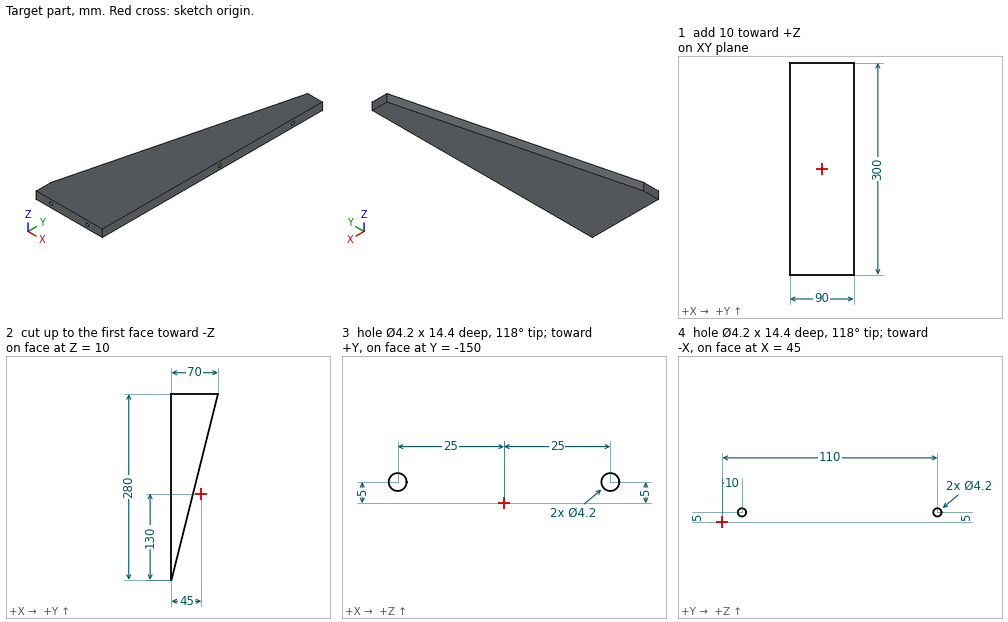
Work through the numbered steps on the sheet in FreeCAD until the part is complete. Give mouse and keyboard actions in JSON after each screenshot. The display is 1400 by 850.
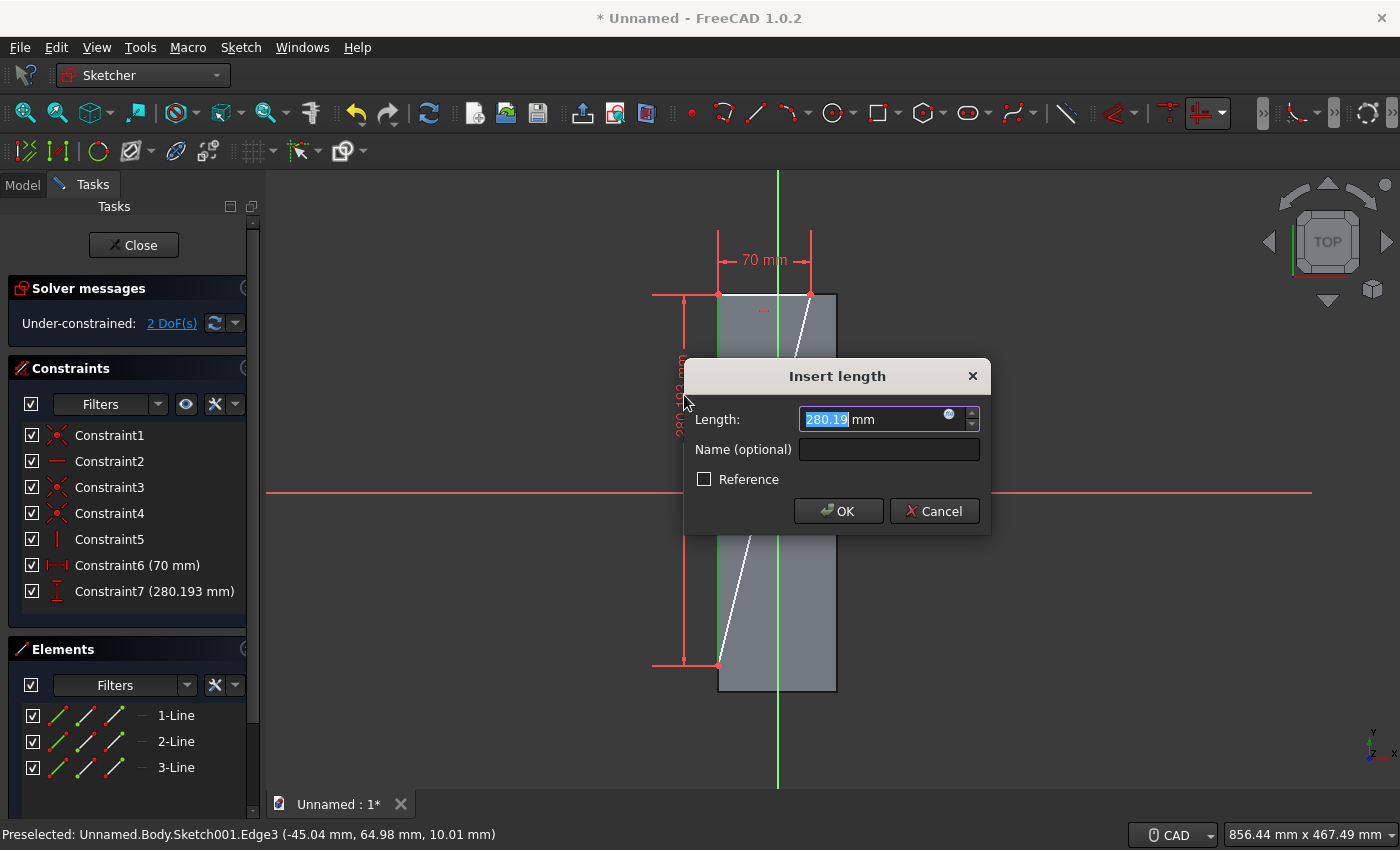
{"action": "type", "text": "280"}
{"action": "key", "text": "Return"}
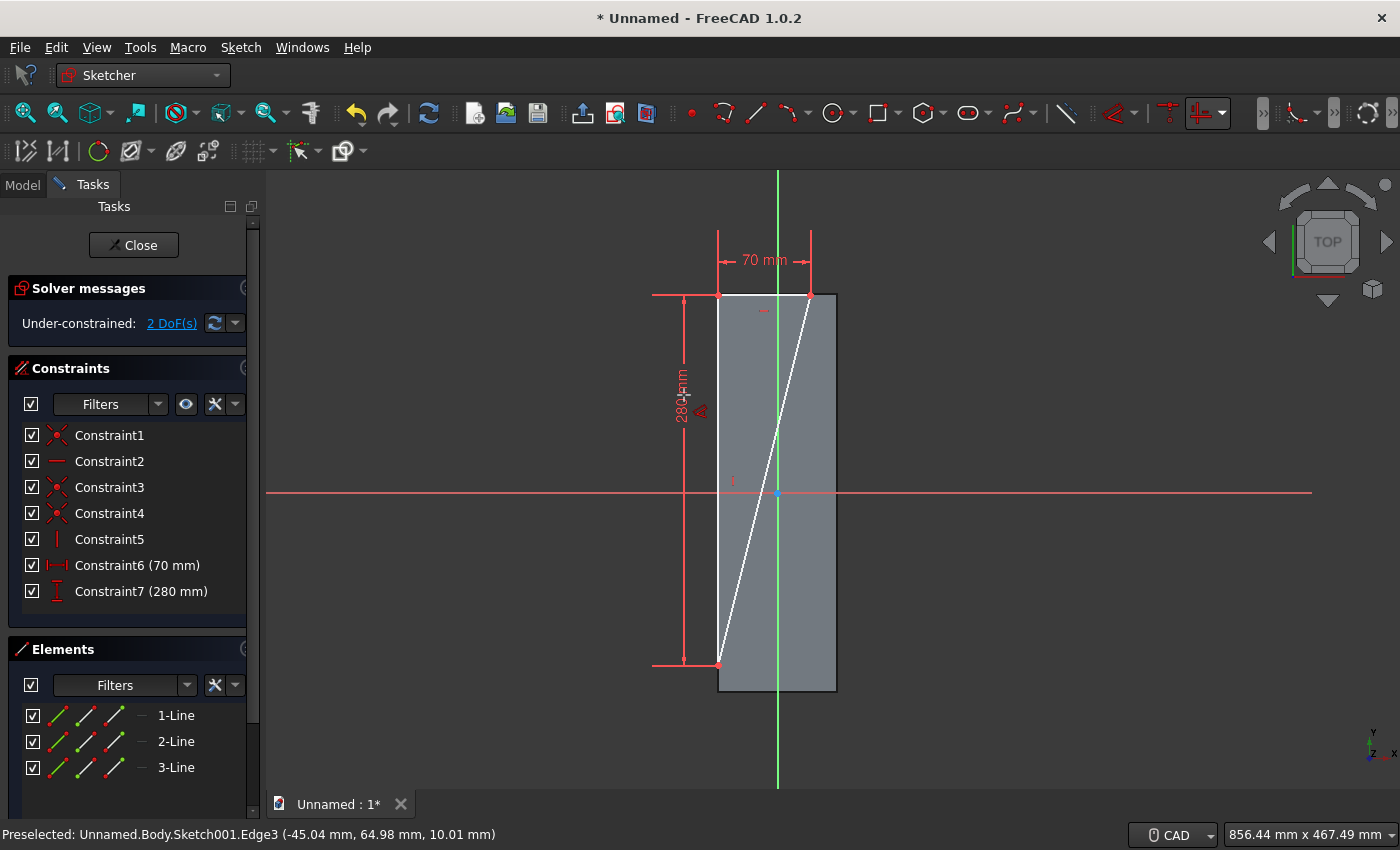
{"action": "left_click", "coordinate": [718, 666]}
{"action": "left_click", "coordinate": [748, 700]}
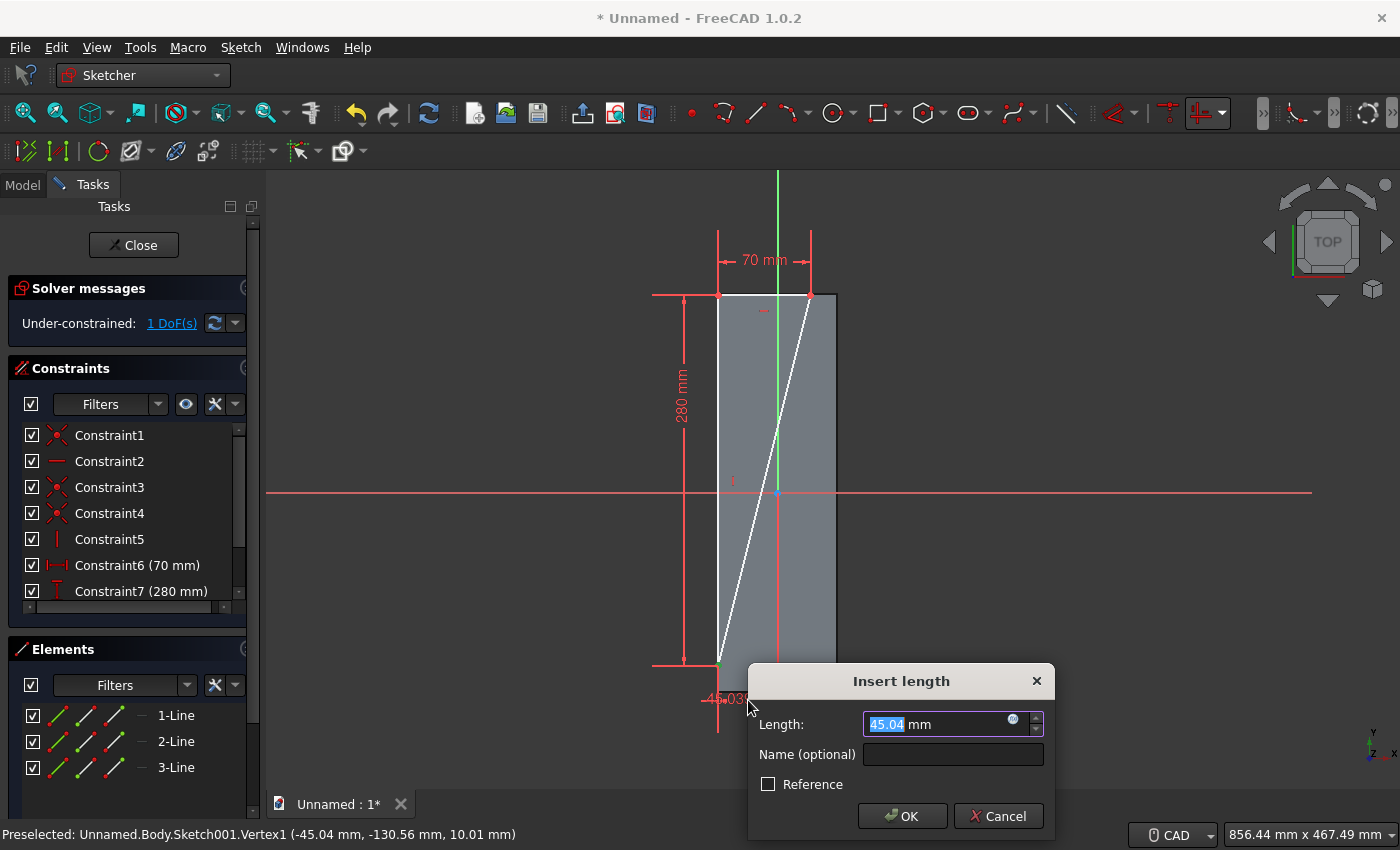
{"action": "type", "text": "45"}
{"action": "key", "text": "Return"}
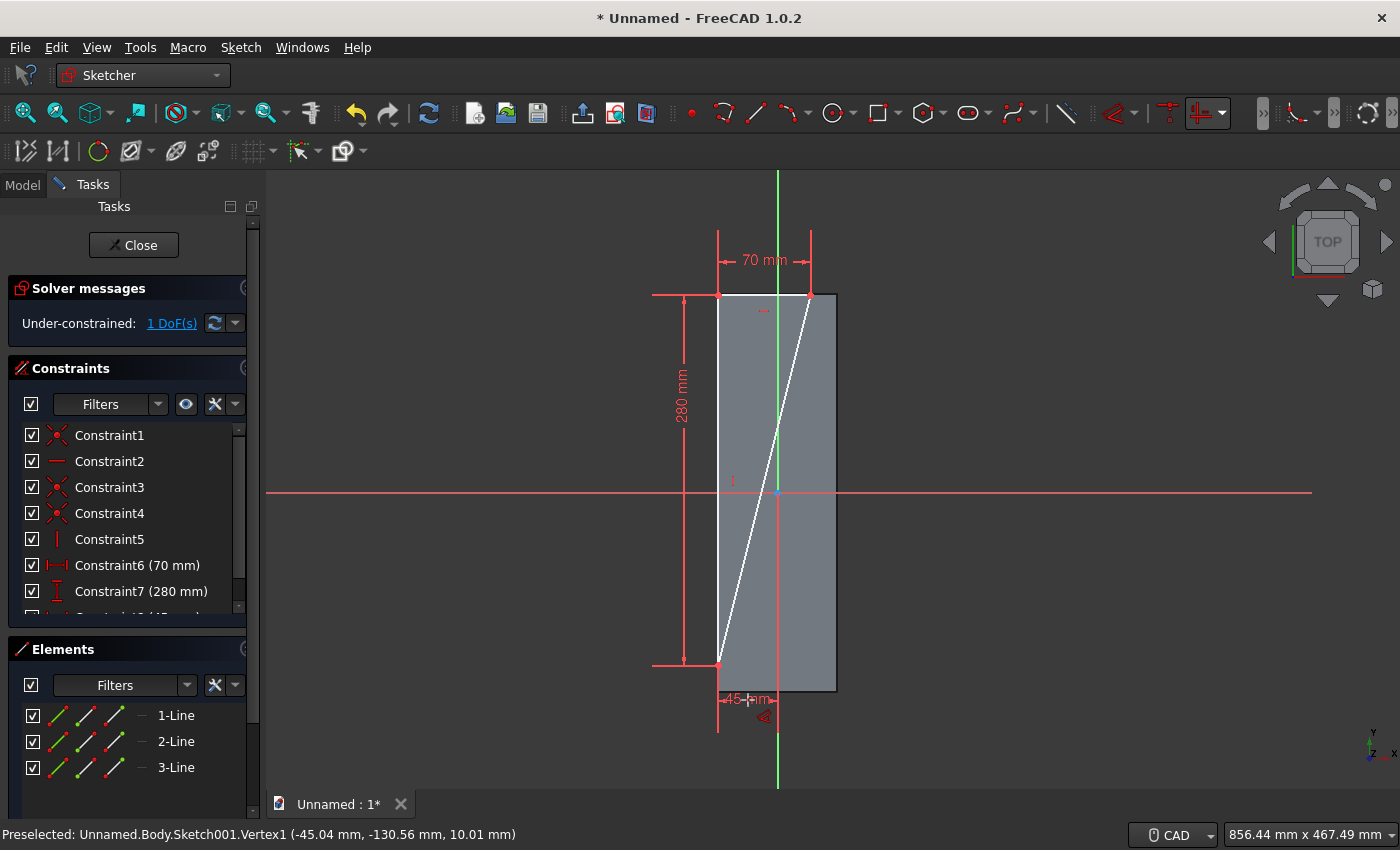
{"action": "left_click", "coordinate": [718, 666]}
{"action": "left_click", "coordinate": [684, 579]}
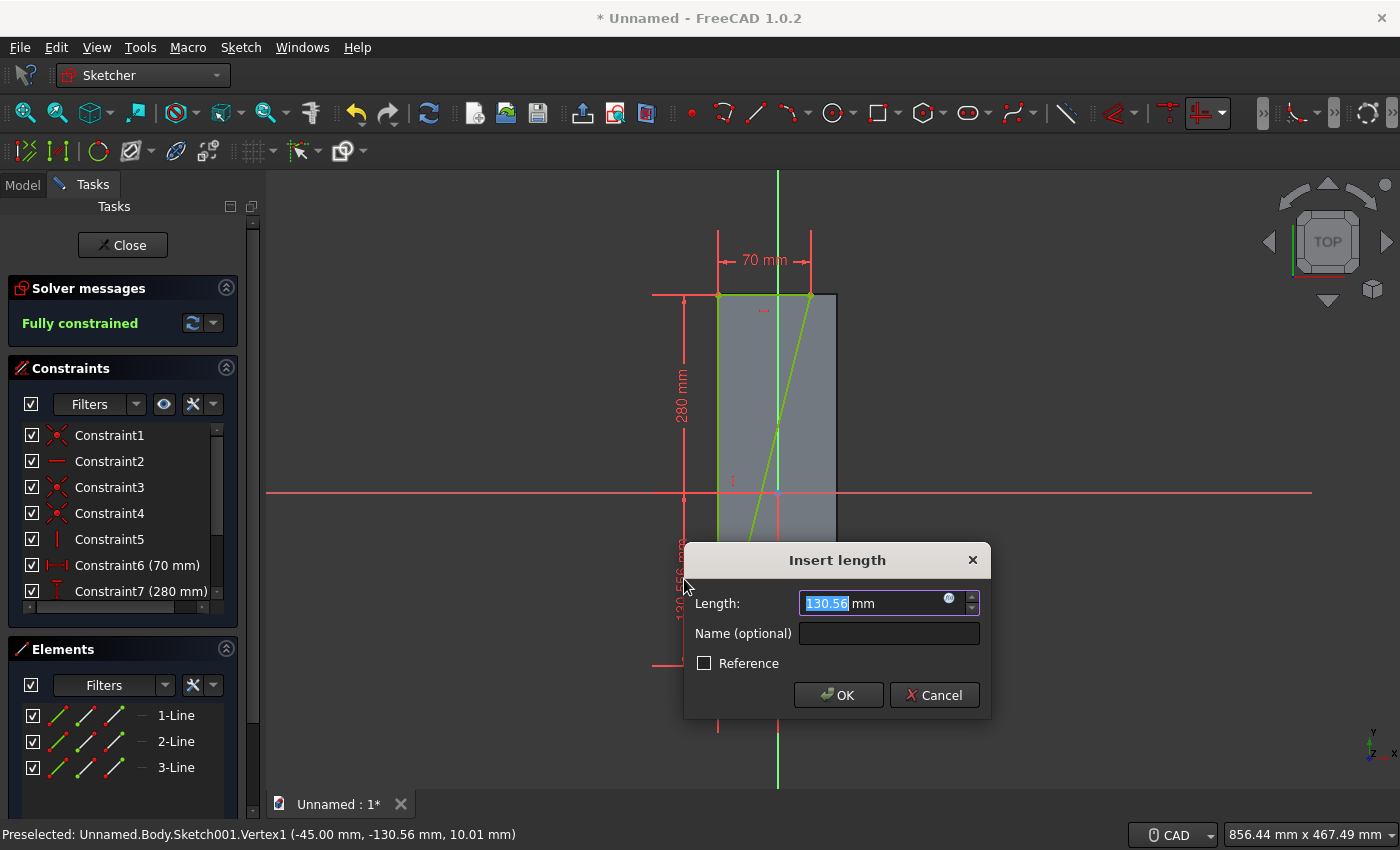
{"action": "type", "text": "130"}
{"action": "key", "text": "Return"}
{"action": "key", "text": "Escape"}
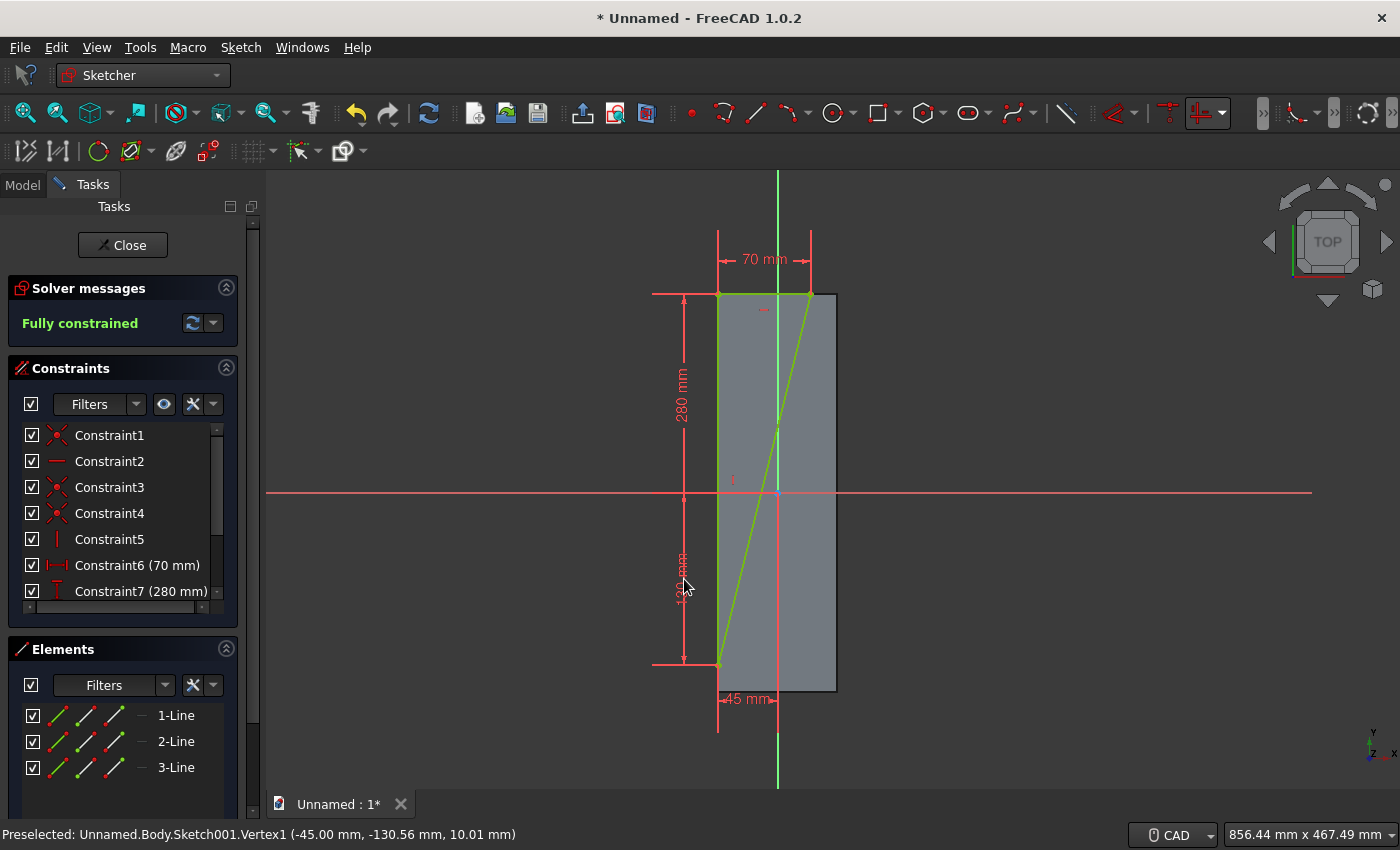
{"action": "left_click", "coordinate": [123, 245]}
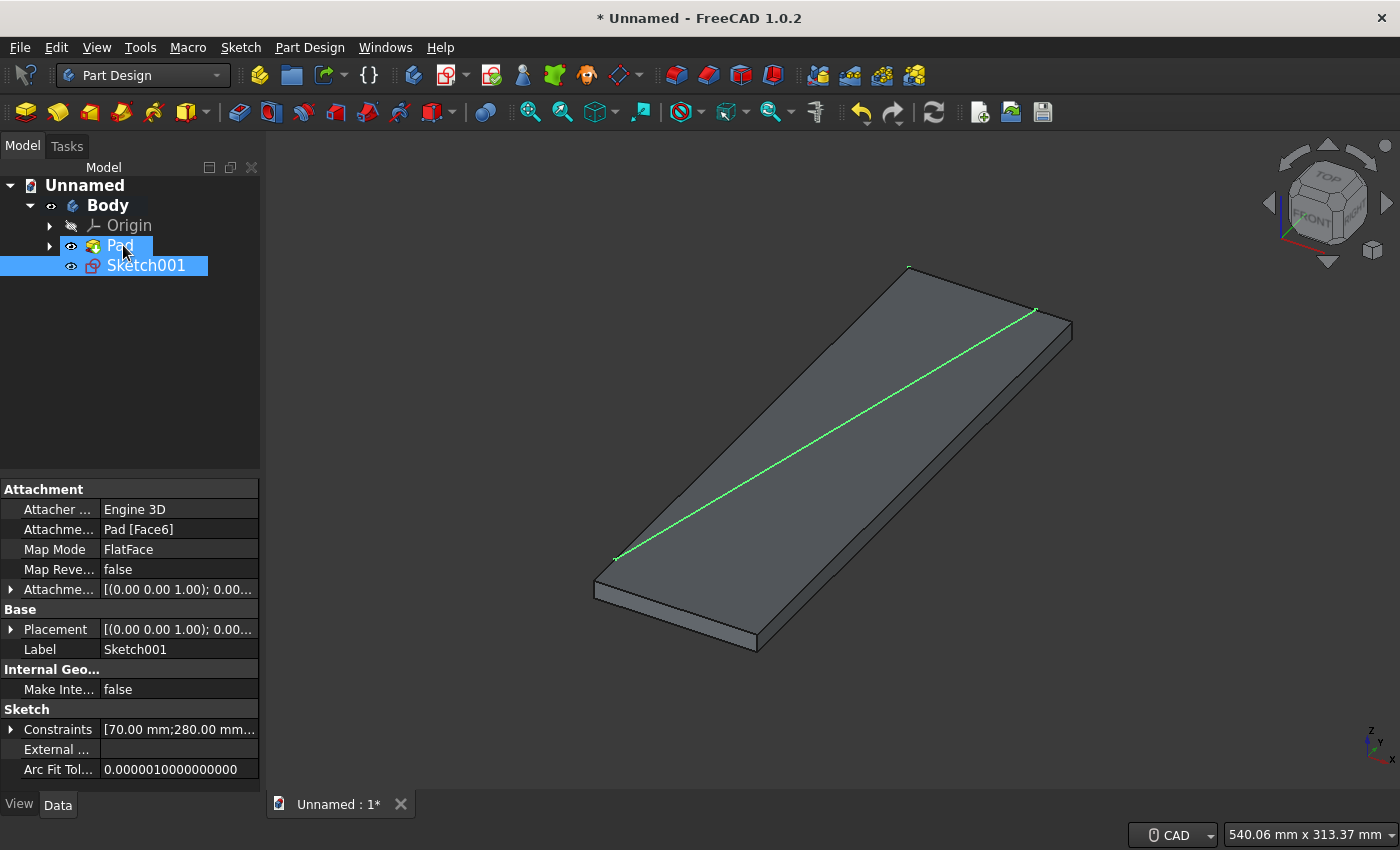
{"action": "left_click", "coordinate": [240, 112]}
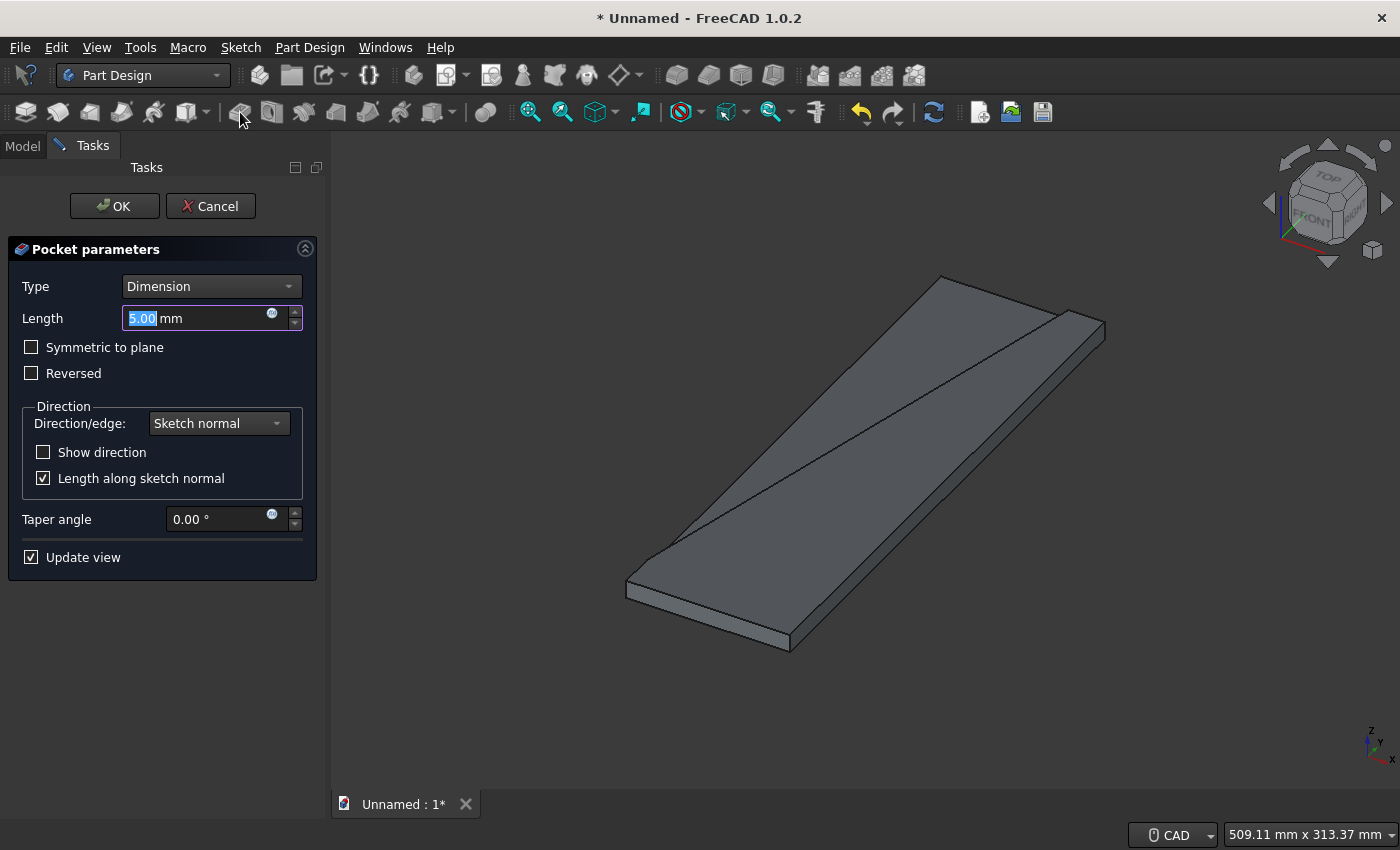
{"action": "left_click", "coordinate": [212, 286]}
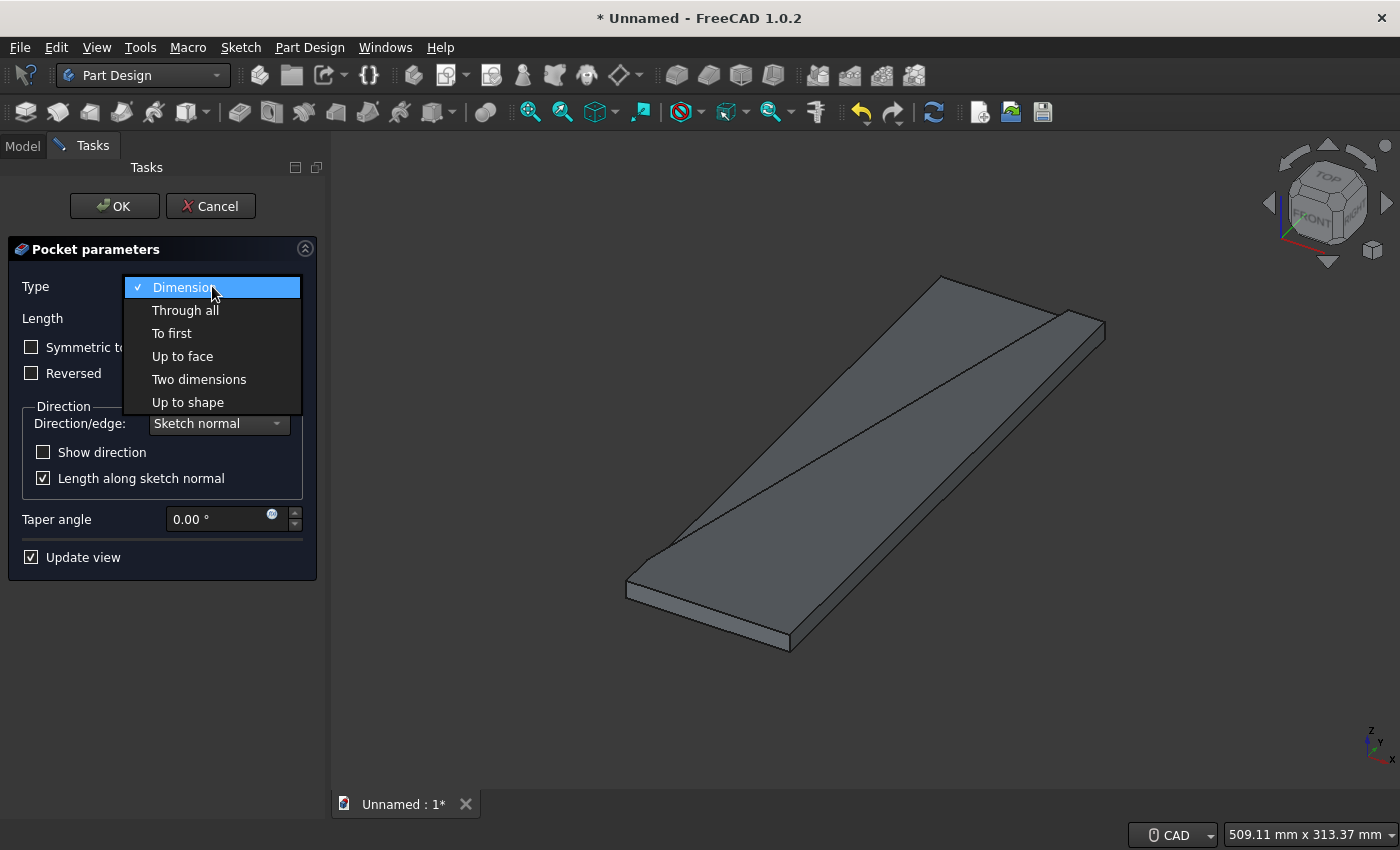
{"action": "left_click", "coordinate": [212, 334]}